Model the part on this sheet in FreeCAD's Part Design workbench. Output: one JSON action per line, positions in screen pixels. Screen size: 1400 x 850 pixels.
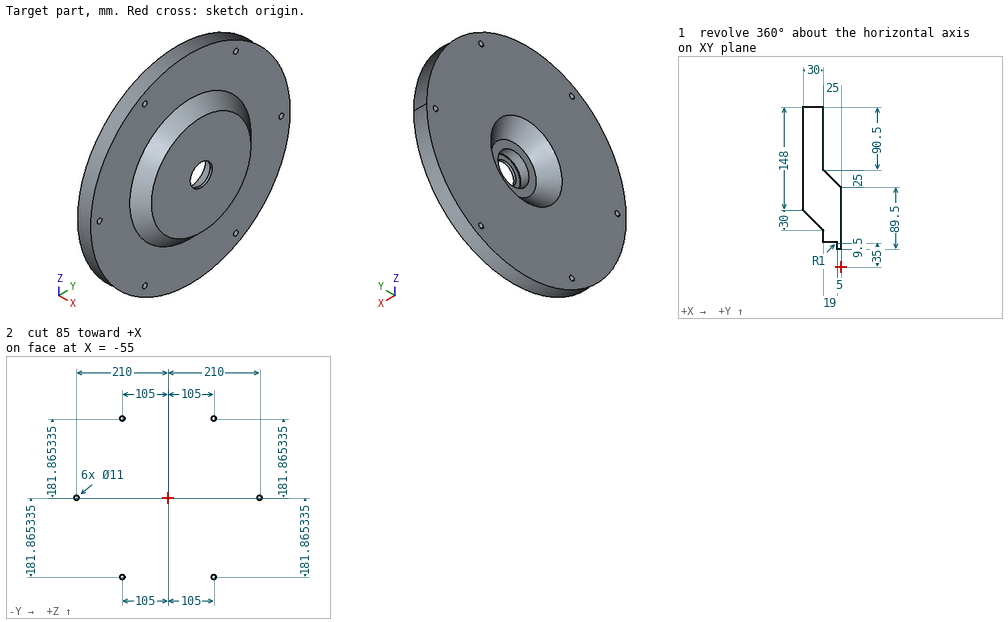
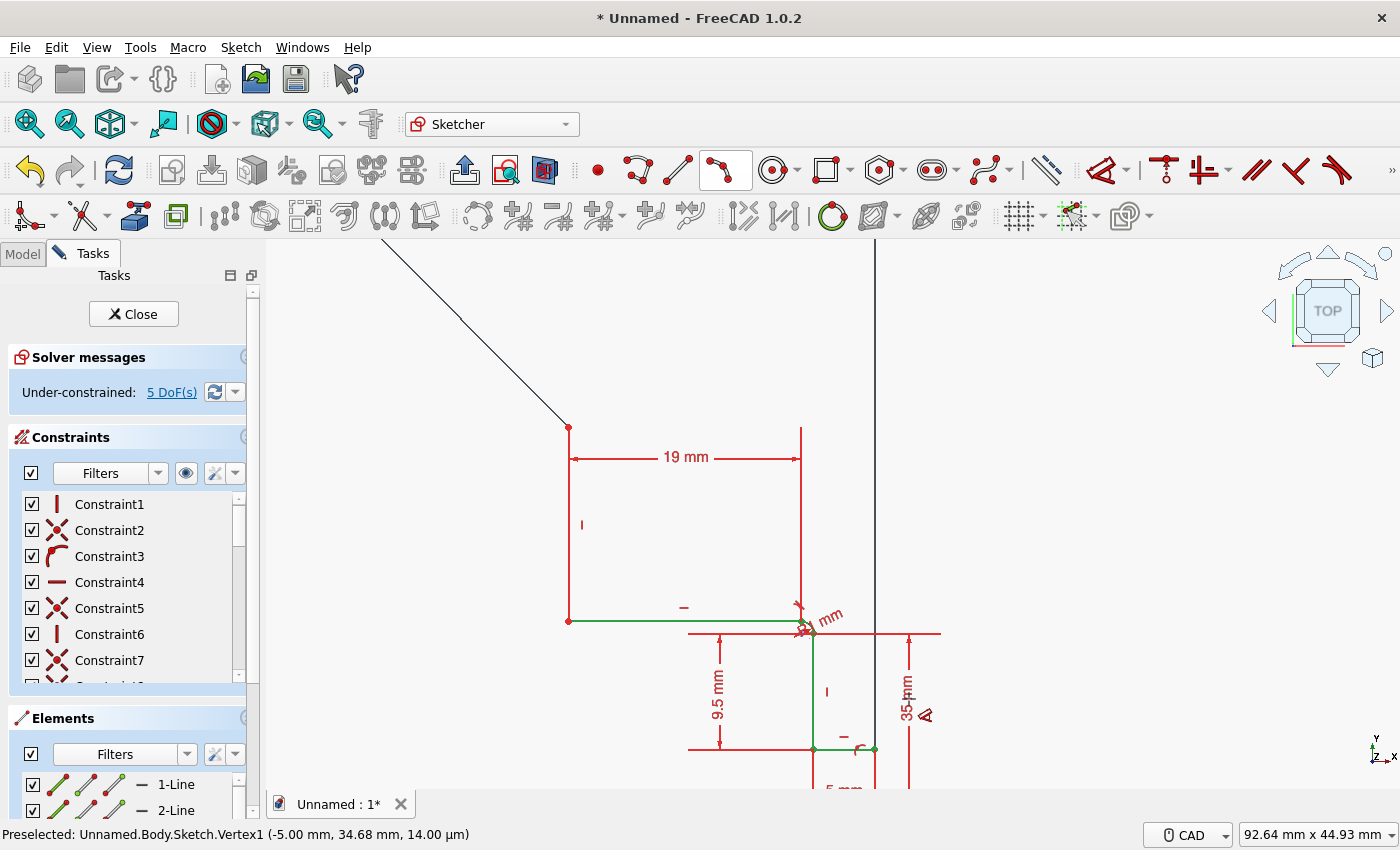
{"action": "scroll", "coordinate": [800, 649], "scroll_direction": "down", "scroll_amount": 10}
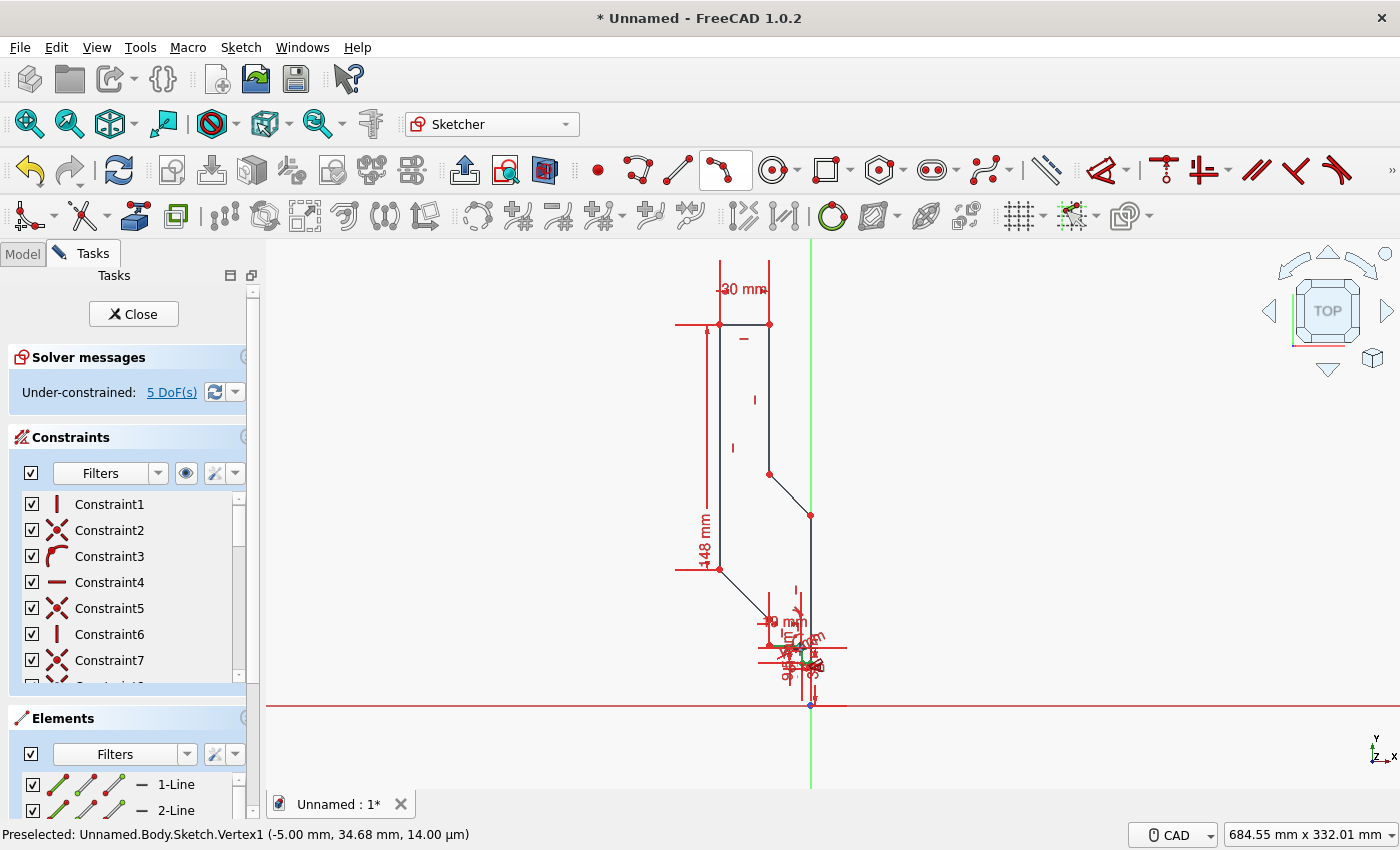
{"action": "left_click", "coordinate": [769, 474]}
{"action": "left_click", "coordinate": [790, 740]}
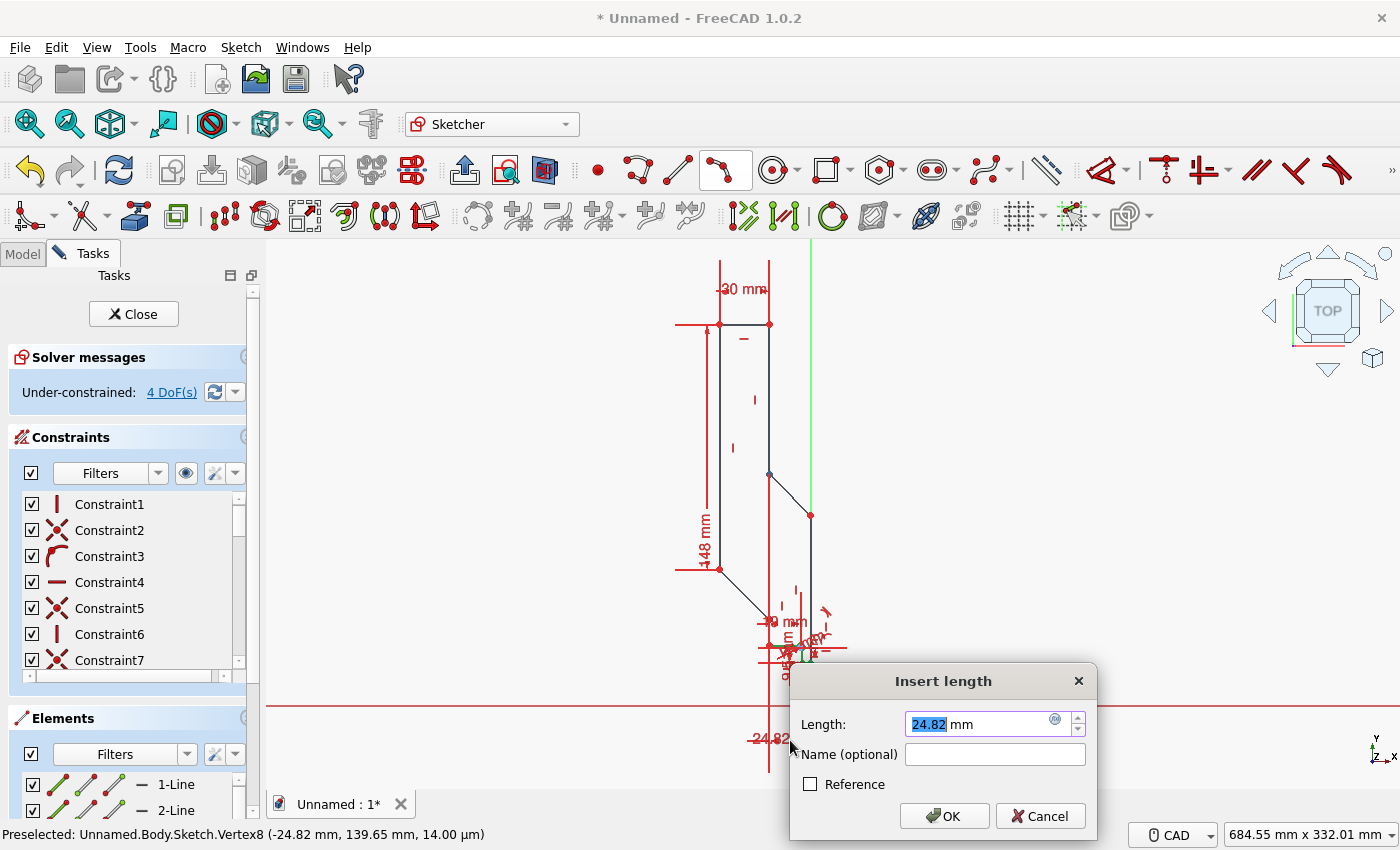
{"action": "type", "text": "25"}
{"action": "key", "text": "Return"}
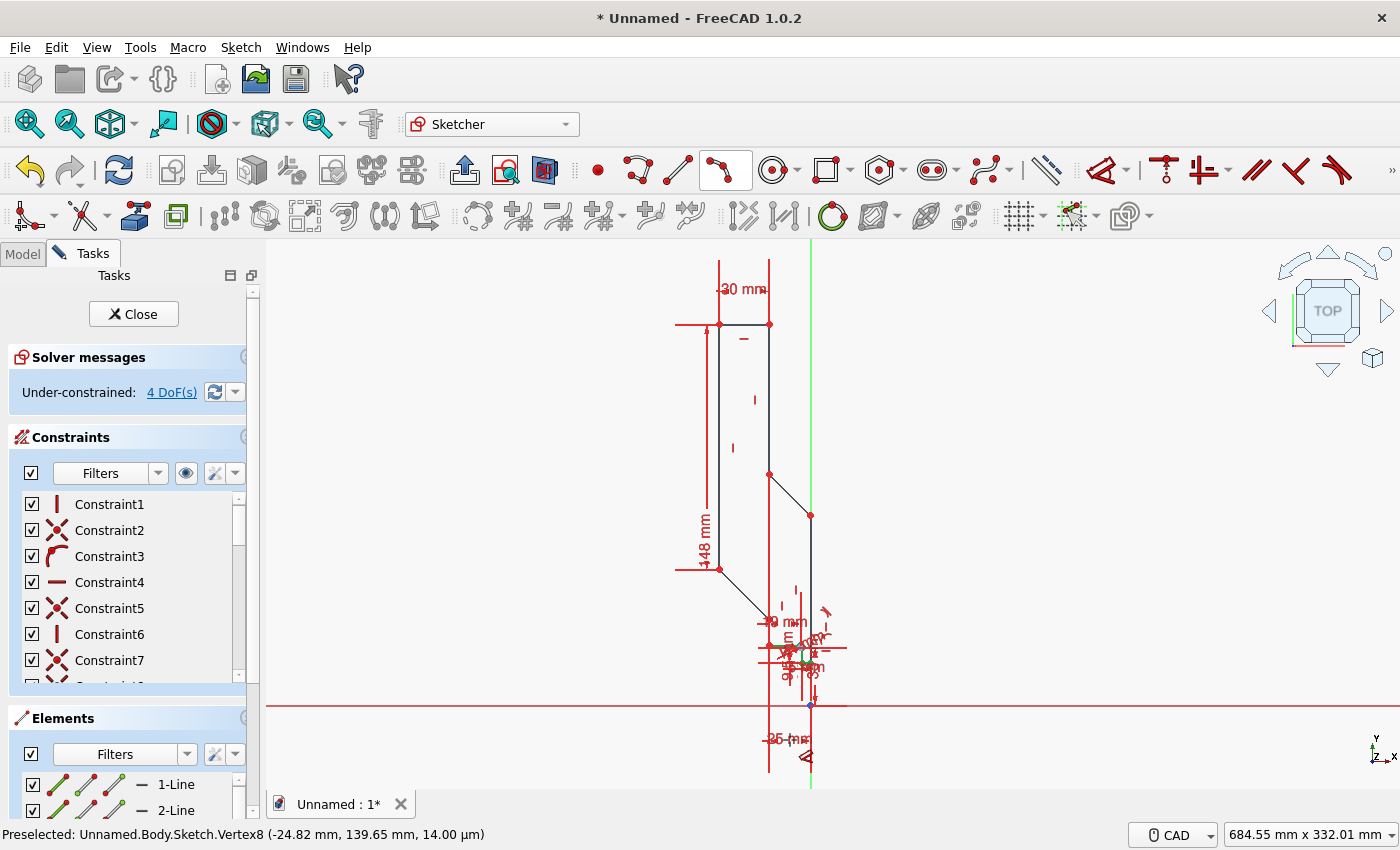
{"action": "left_click", "coordinate": [798, 503]}
{"action": "left_click", "coordinate": [845, 495]}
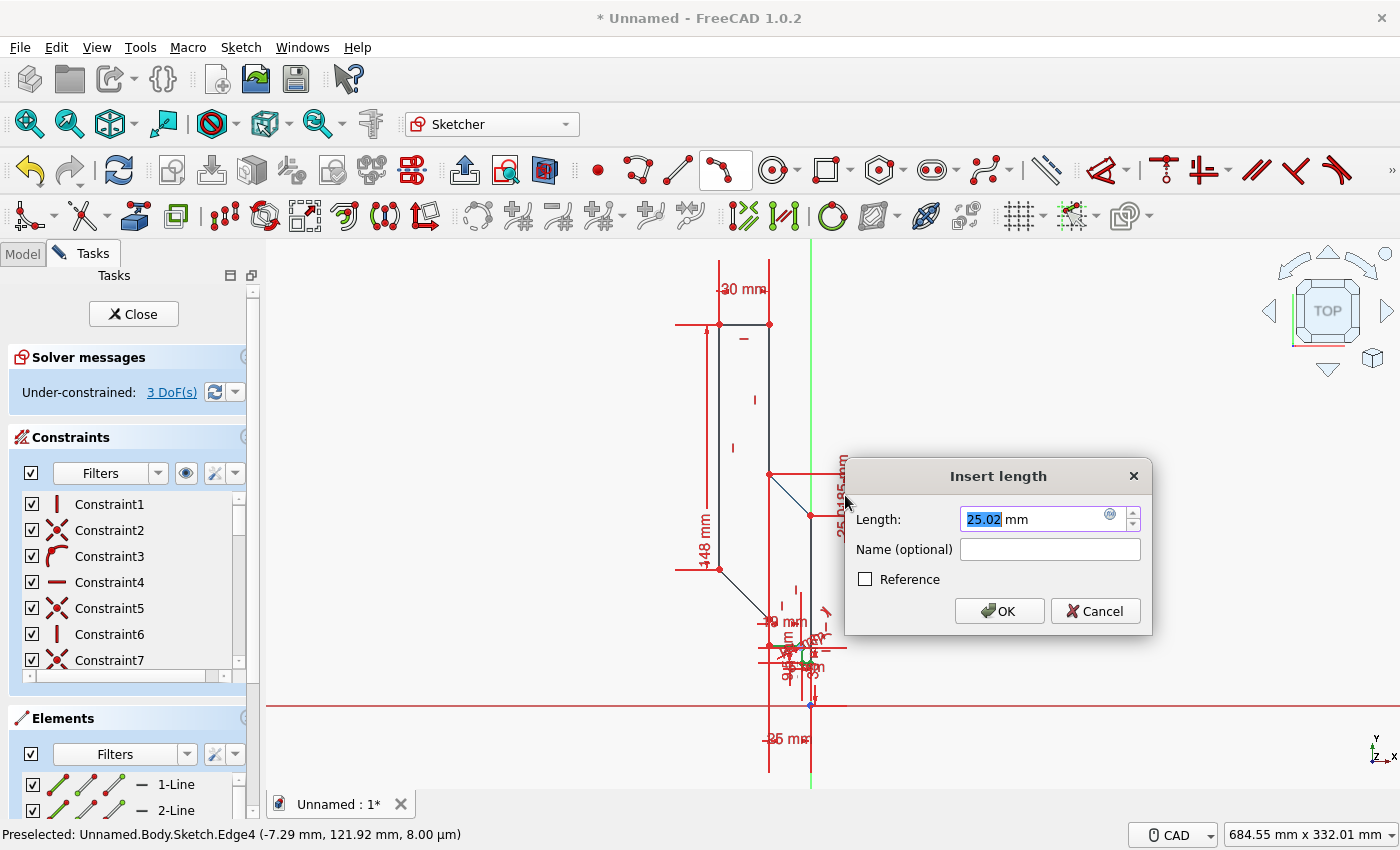
{"action": "type", "text": "25"}
{"action": "key", "text": "Return"}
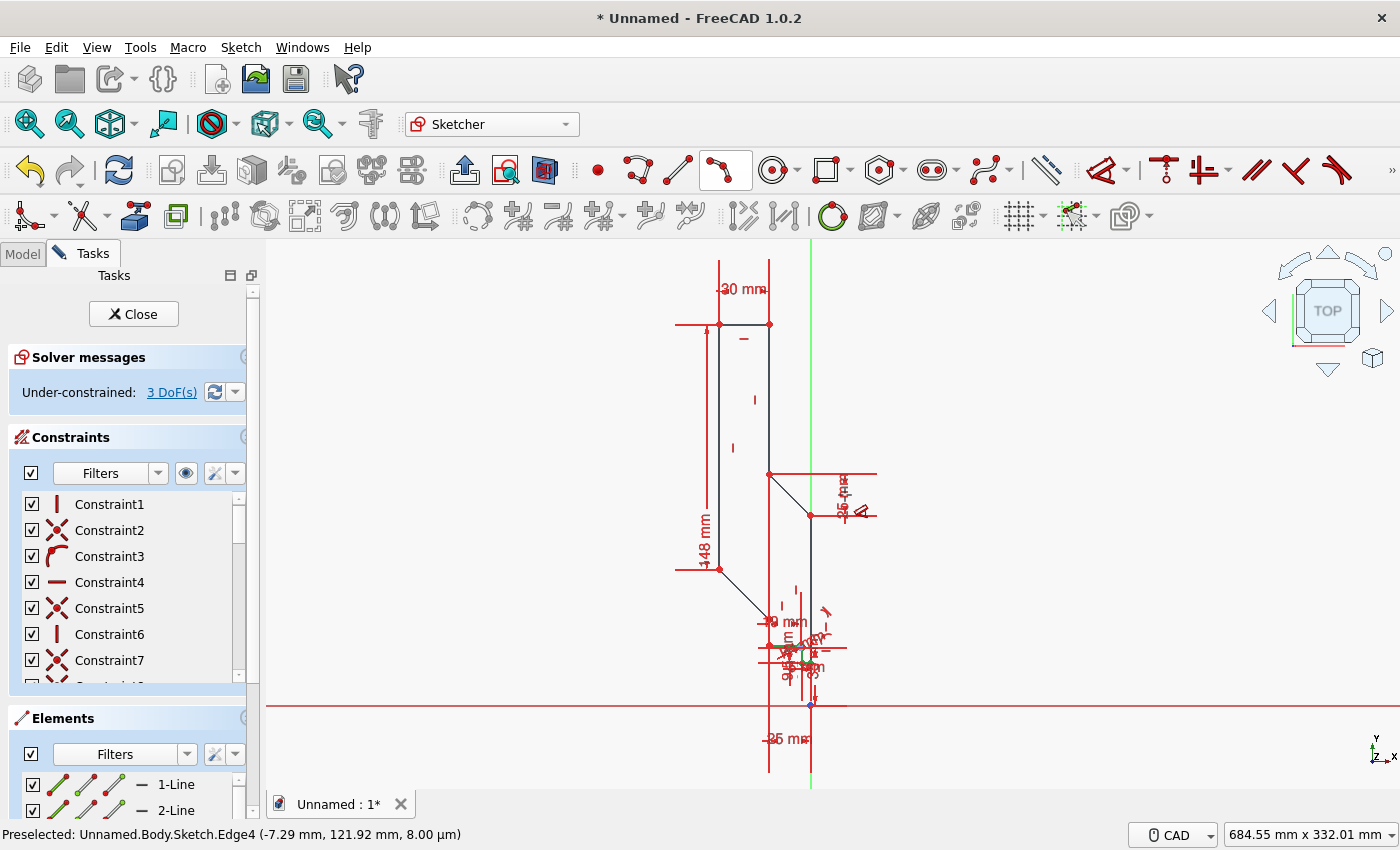
{"action": "left_click", "coordinate": [734, 585]}
{"action": "left_click", "coordinate": [685, 595]}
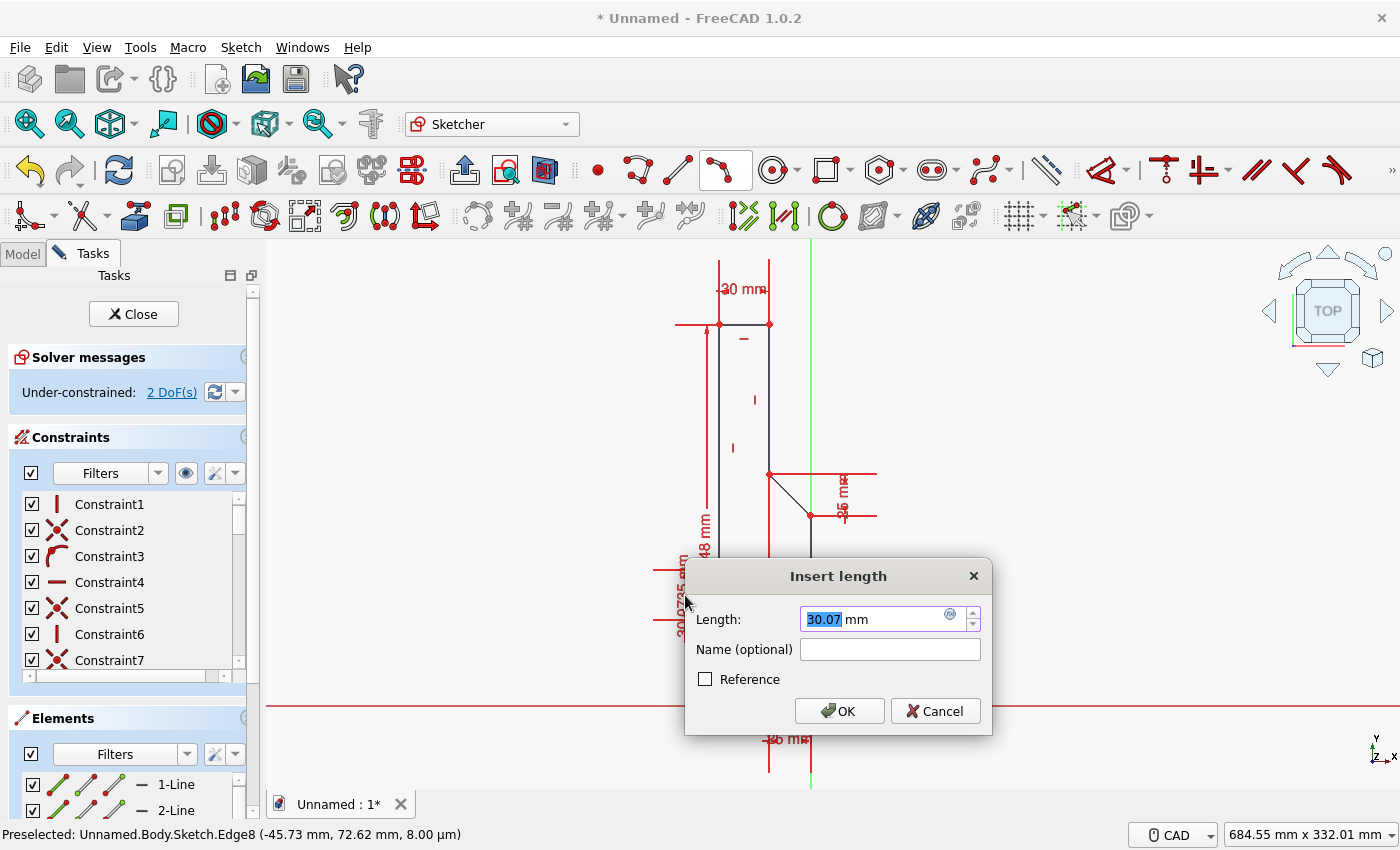
{"action": "type", "text": "30"}
{"action": "key", "text": "Return"}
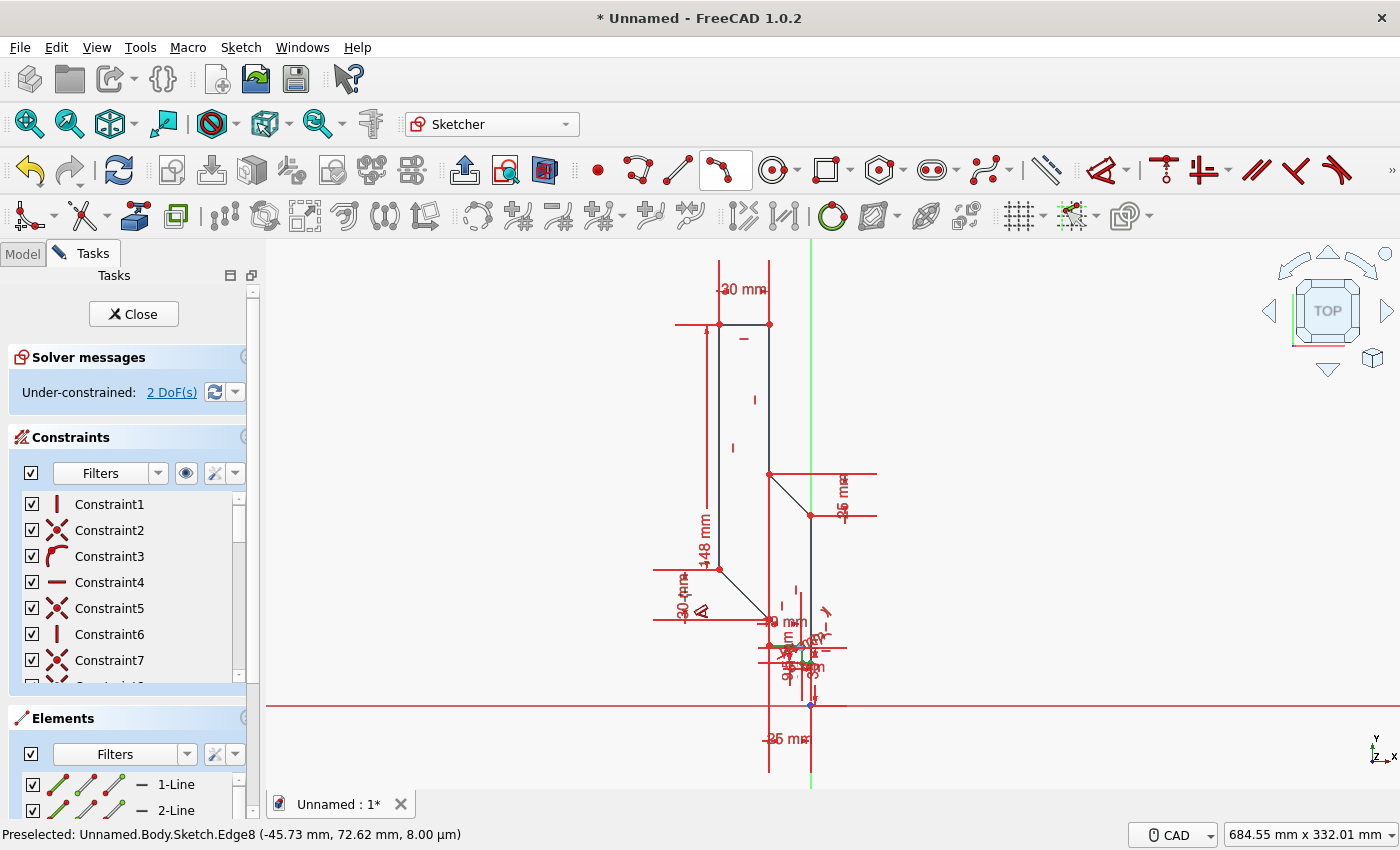
{"action": "left_click", "coordinate": [811, 619]}
{"action": "left_click", "coordinate": [845, 589]}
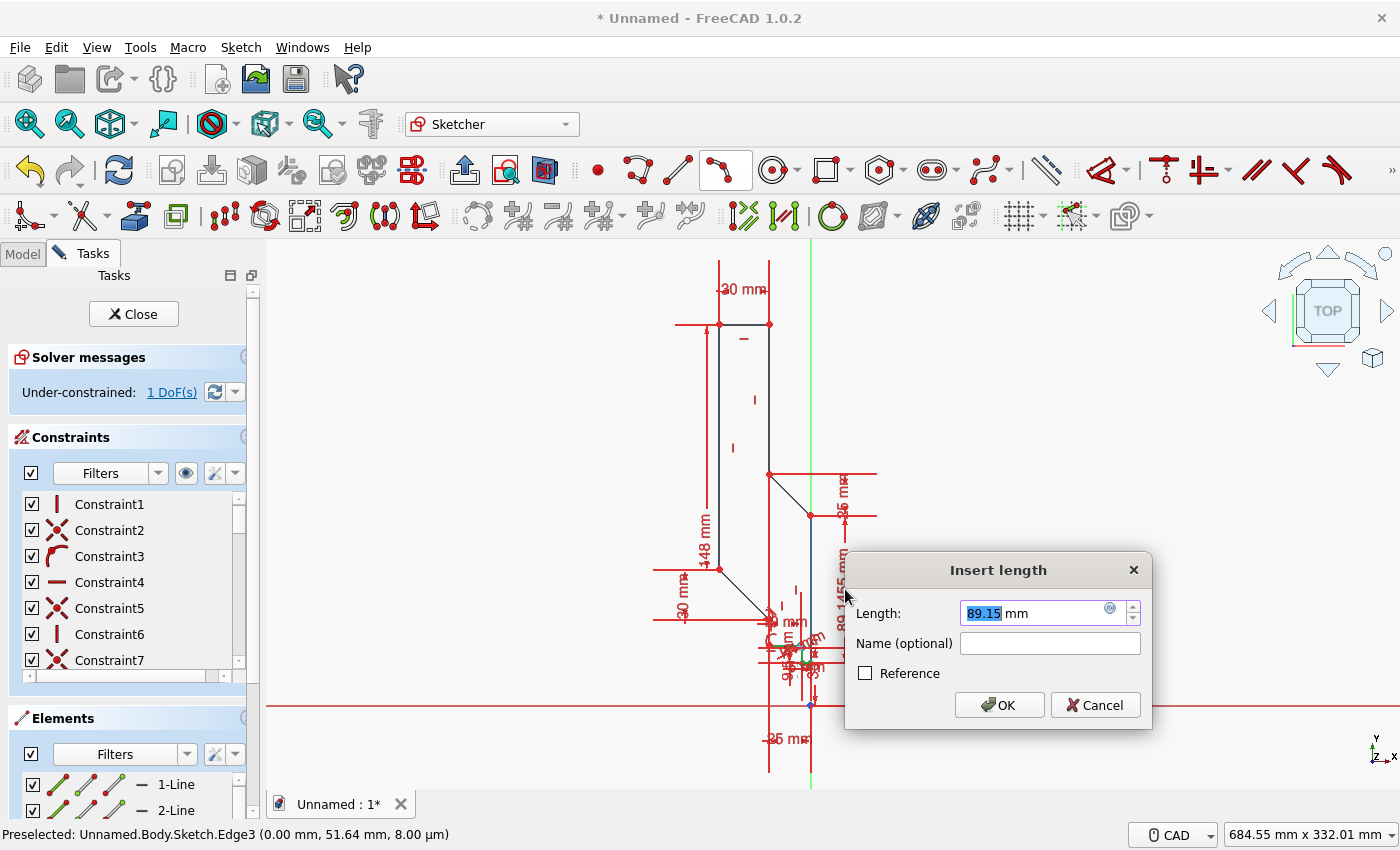
{"action": "type", "text": "89.5"}
{"action": "key", "text": "Return"}